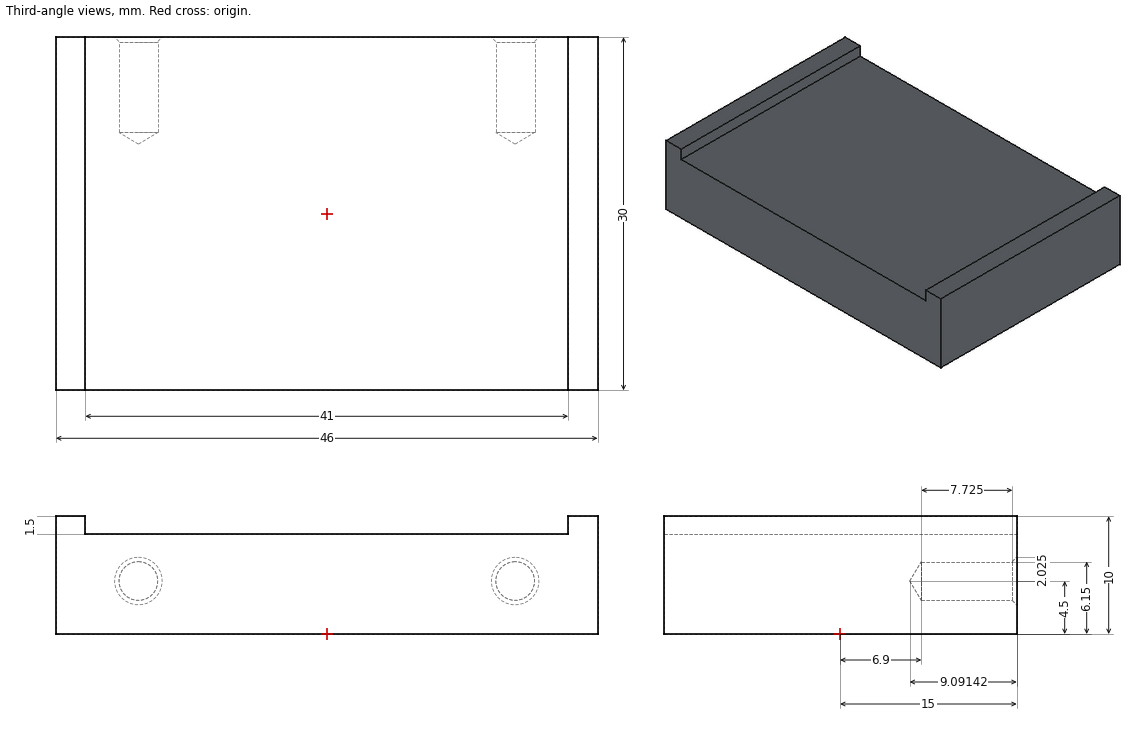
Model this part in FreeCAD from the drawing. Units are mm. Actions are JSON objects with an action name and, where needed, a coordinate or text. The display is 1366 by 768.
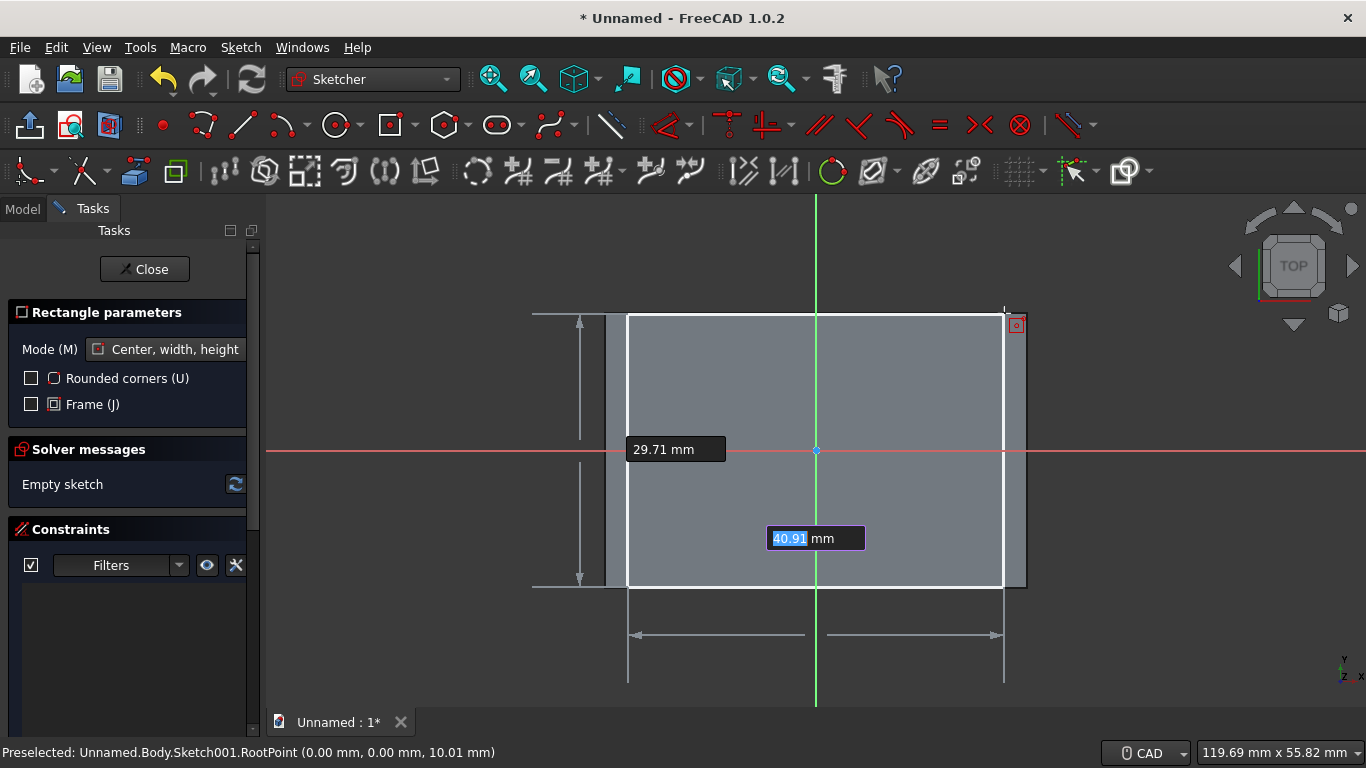
{"action": "type", "text": "41"}
{"action": "key", "text": "Tab"}
{"action": "type", "text": "30"}
{"action": "key", "text": "Return"}
{"action": "key", "text": "Escape"}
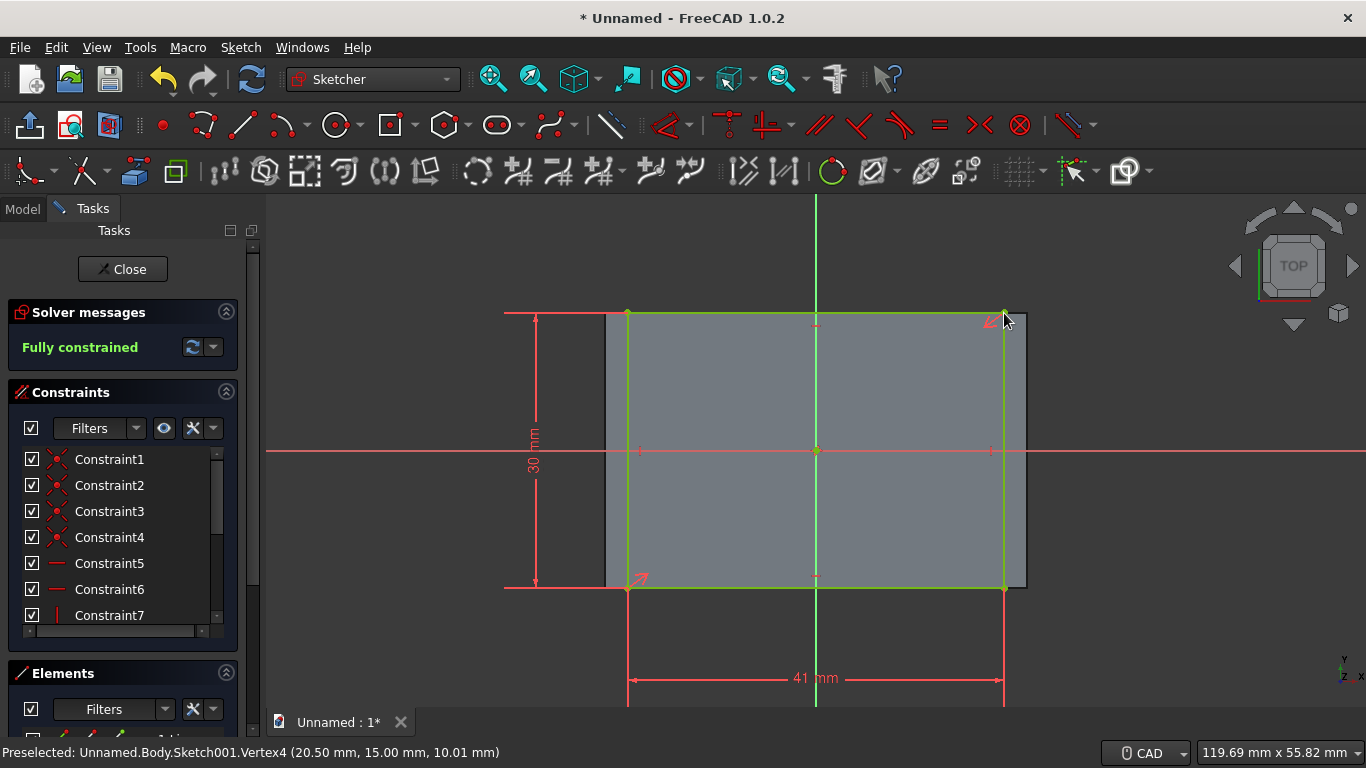
{"action": "left_click", "coordinate": [123, 269]}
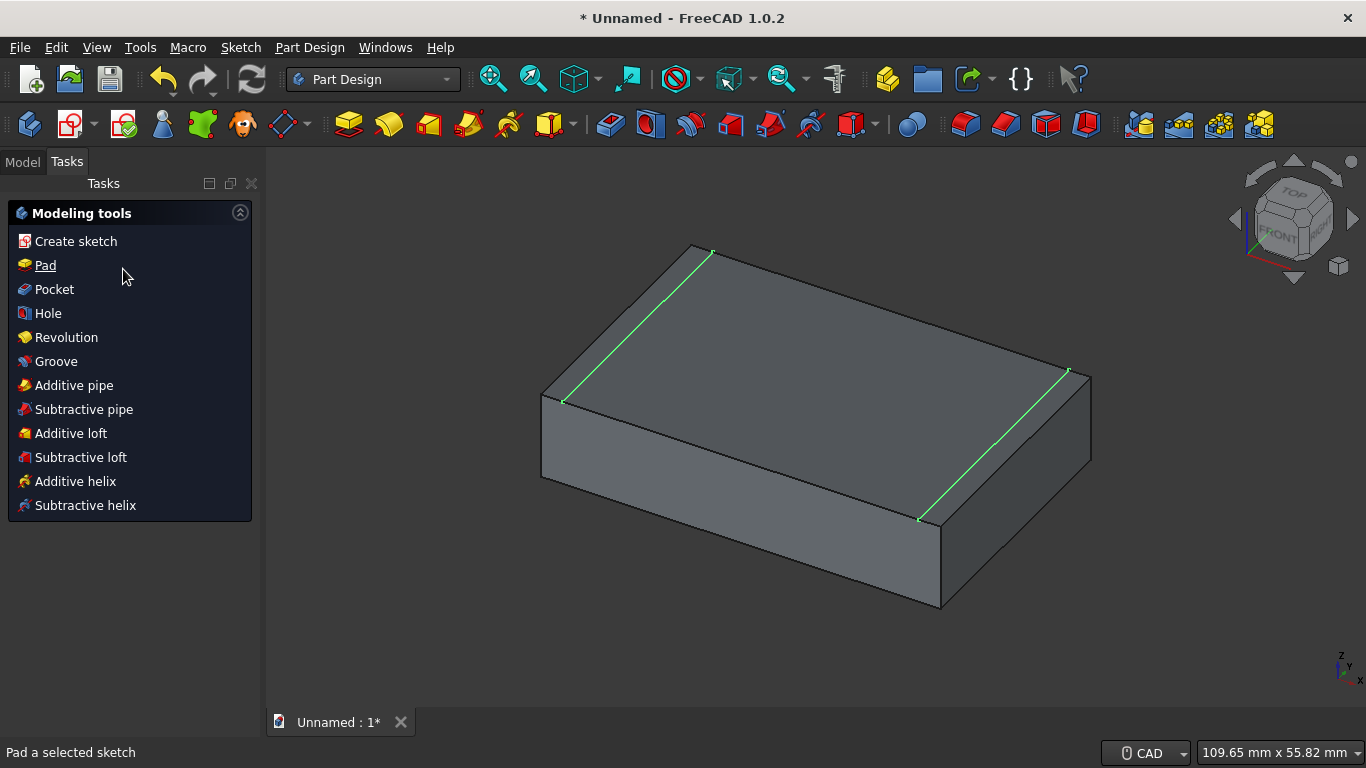
{"action": "left_click", "coordinate": [612, 124]}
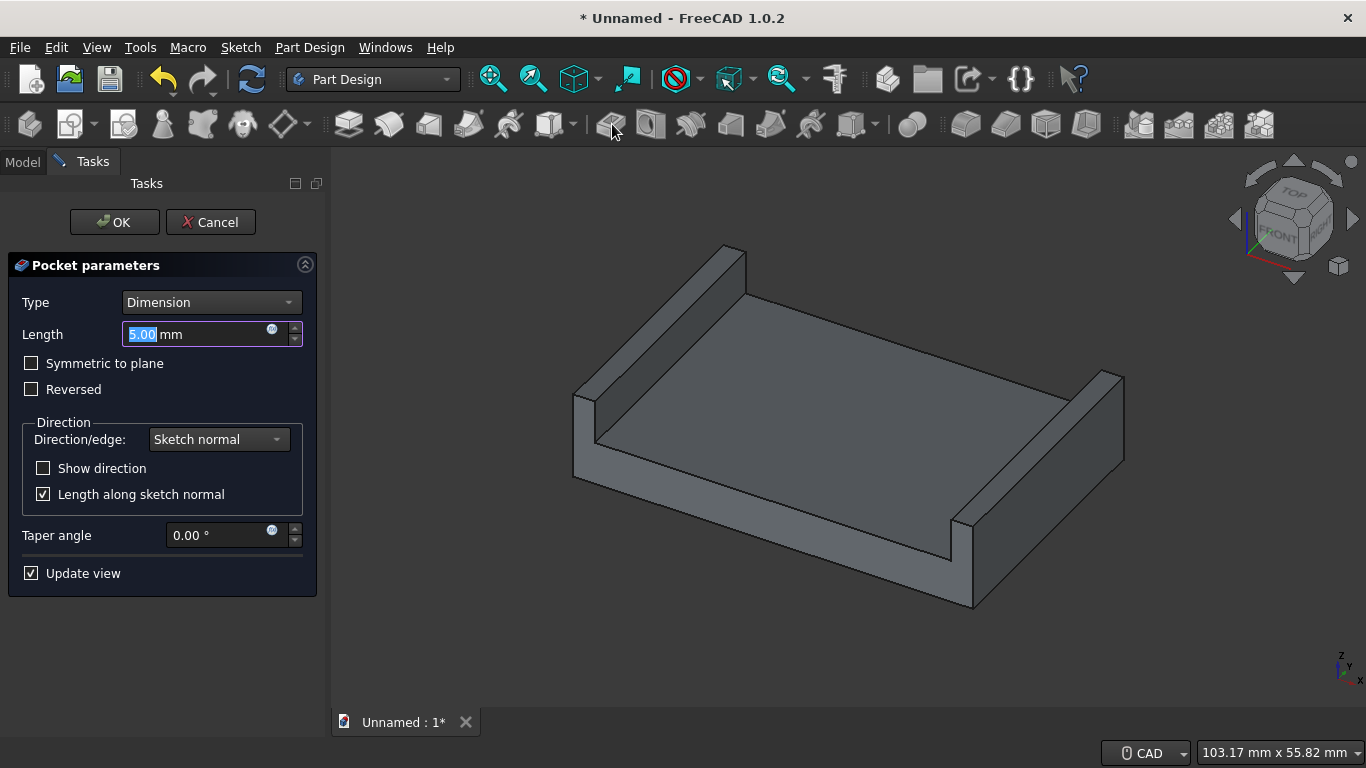
{"action": "type", "text": "1.5"}
{"action": "key", "text": "Tab"}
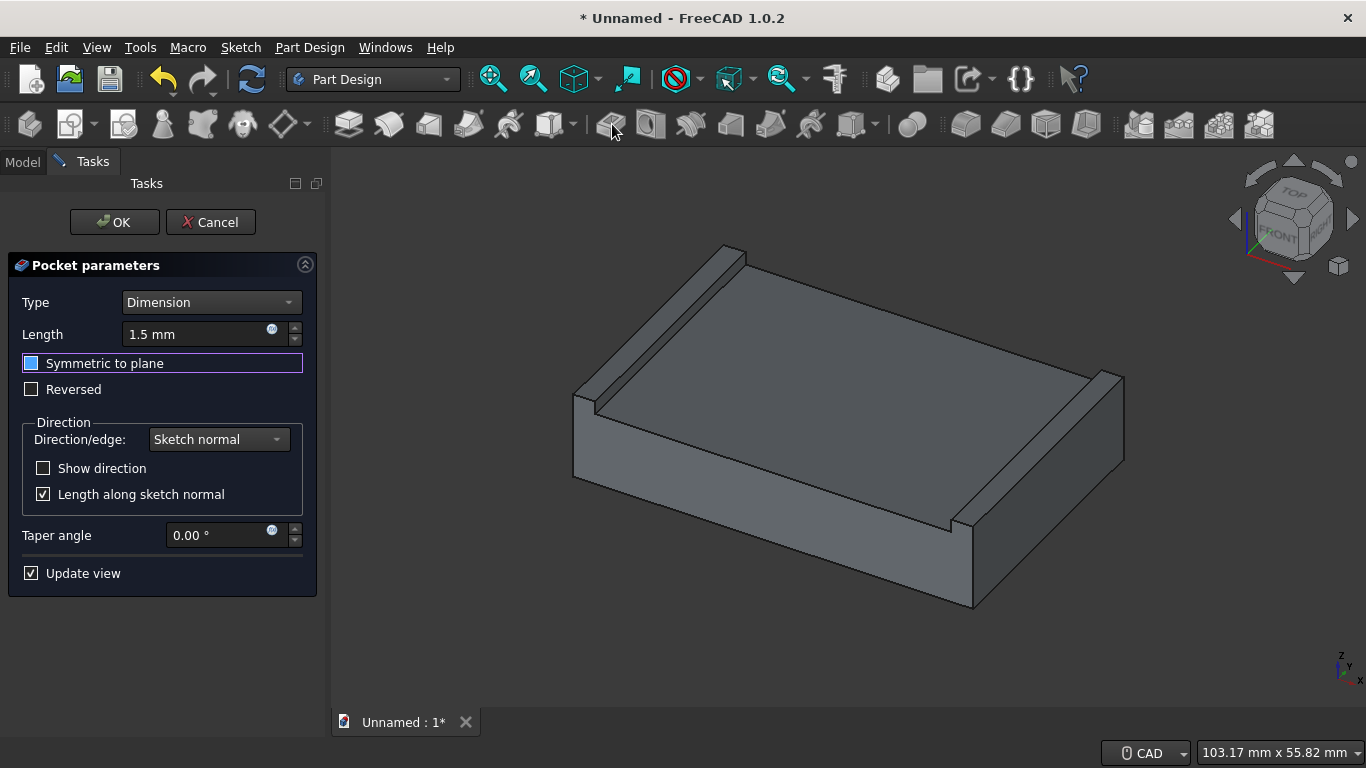
{"action": "left_click", "coordinate": [115, 222]}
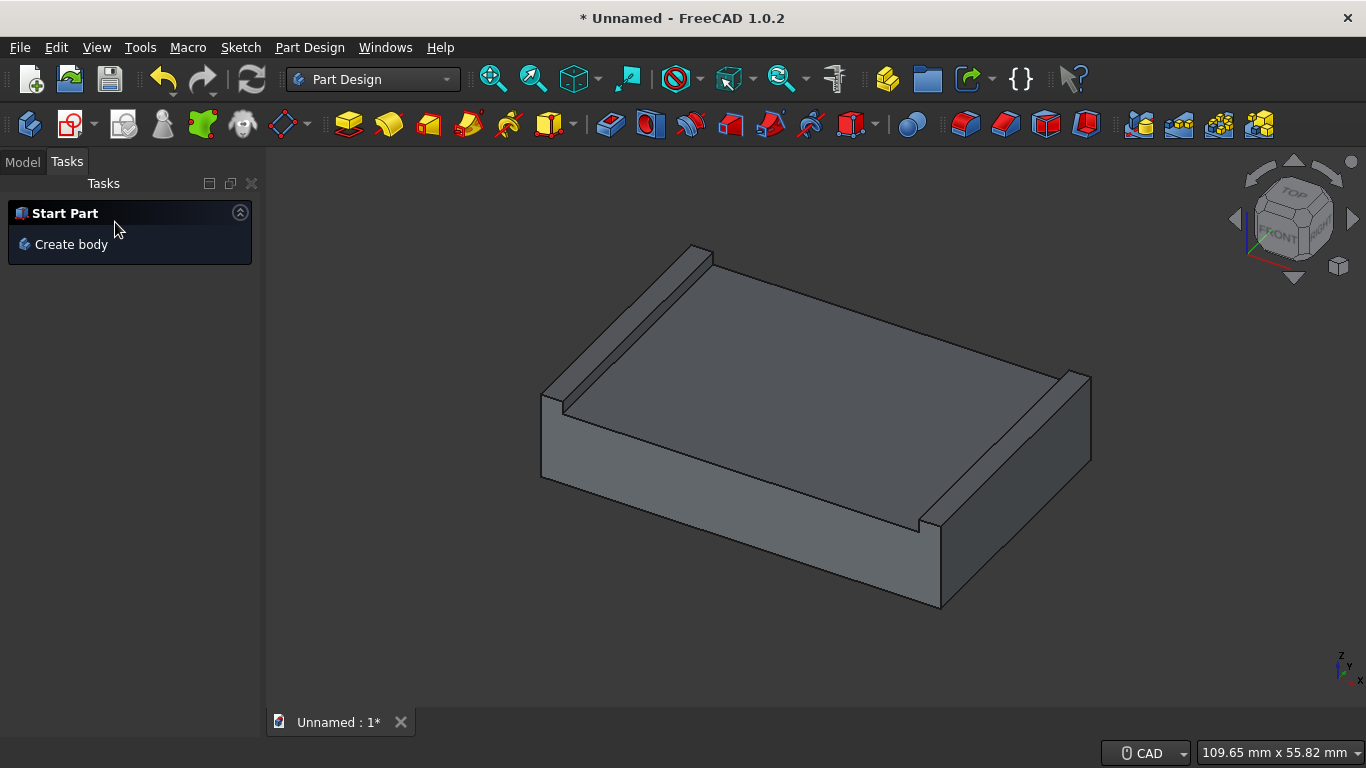
{"action": "left_click", "coordinate": [23, 161]}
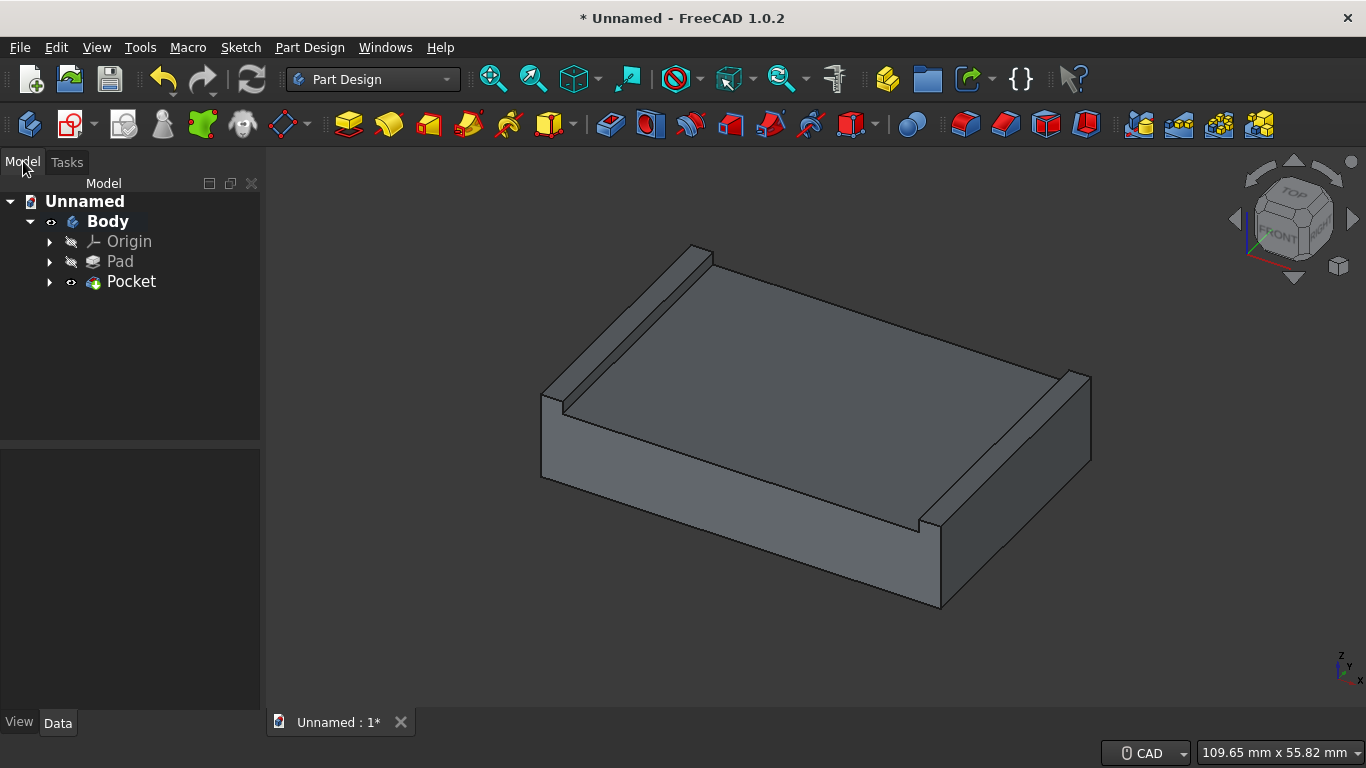
{"action": "left_click", "coordinate": [50, 242]}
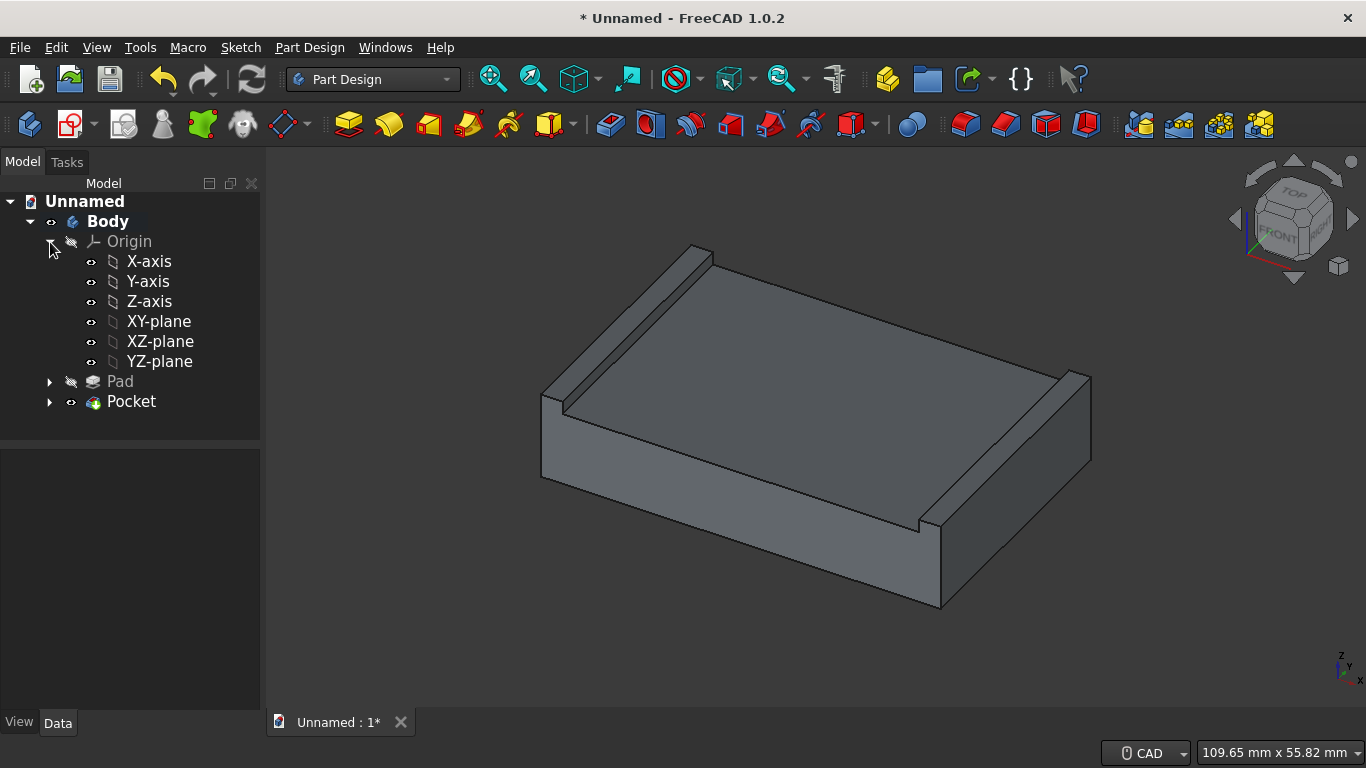
{"action": "left_click", "coordinate": [136, 362]}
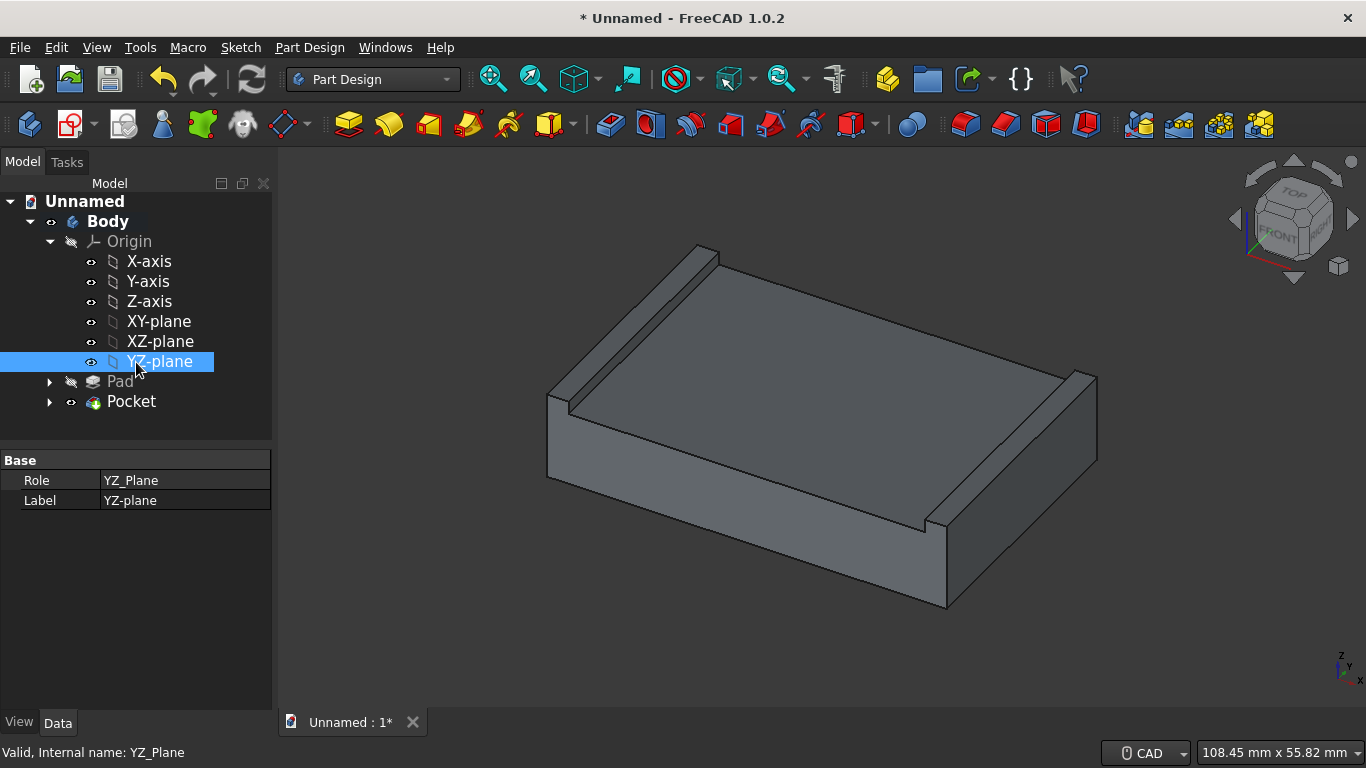
{"action": "left_click", "coordinate": [284, 124]}